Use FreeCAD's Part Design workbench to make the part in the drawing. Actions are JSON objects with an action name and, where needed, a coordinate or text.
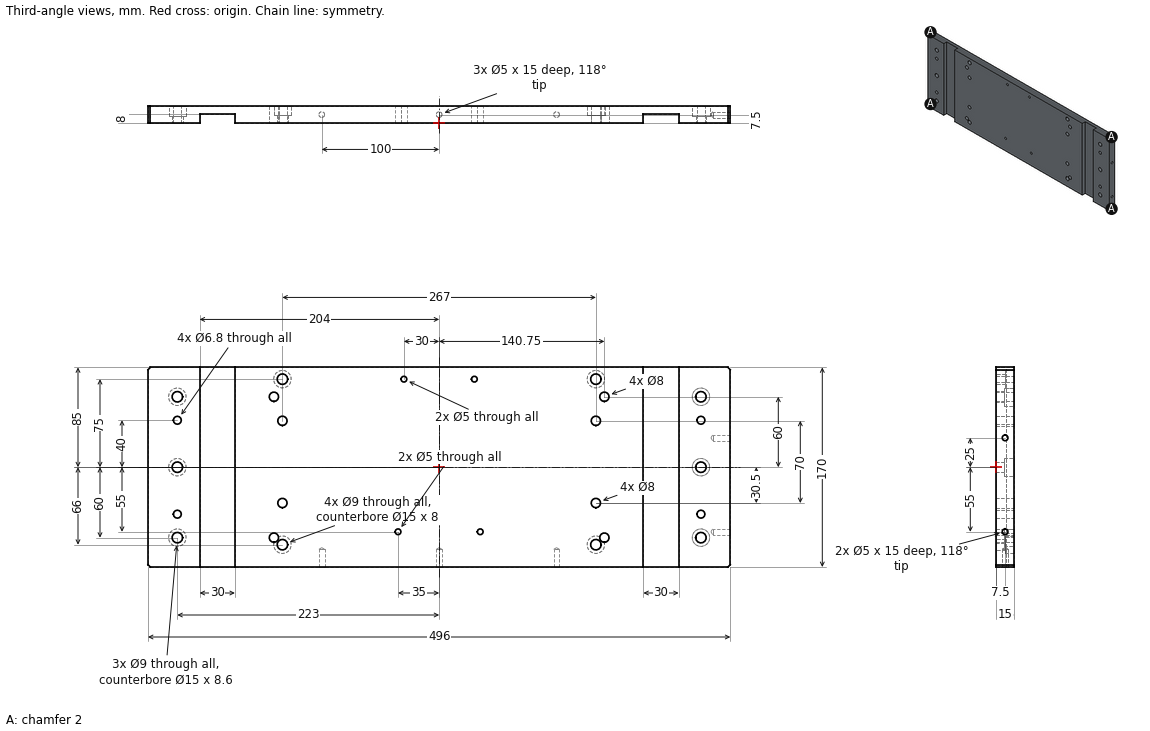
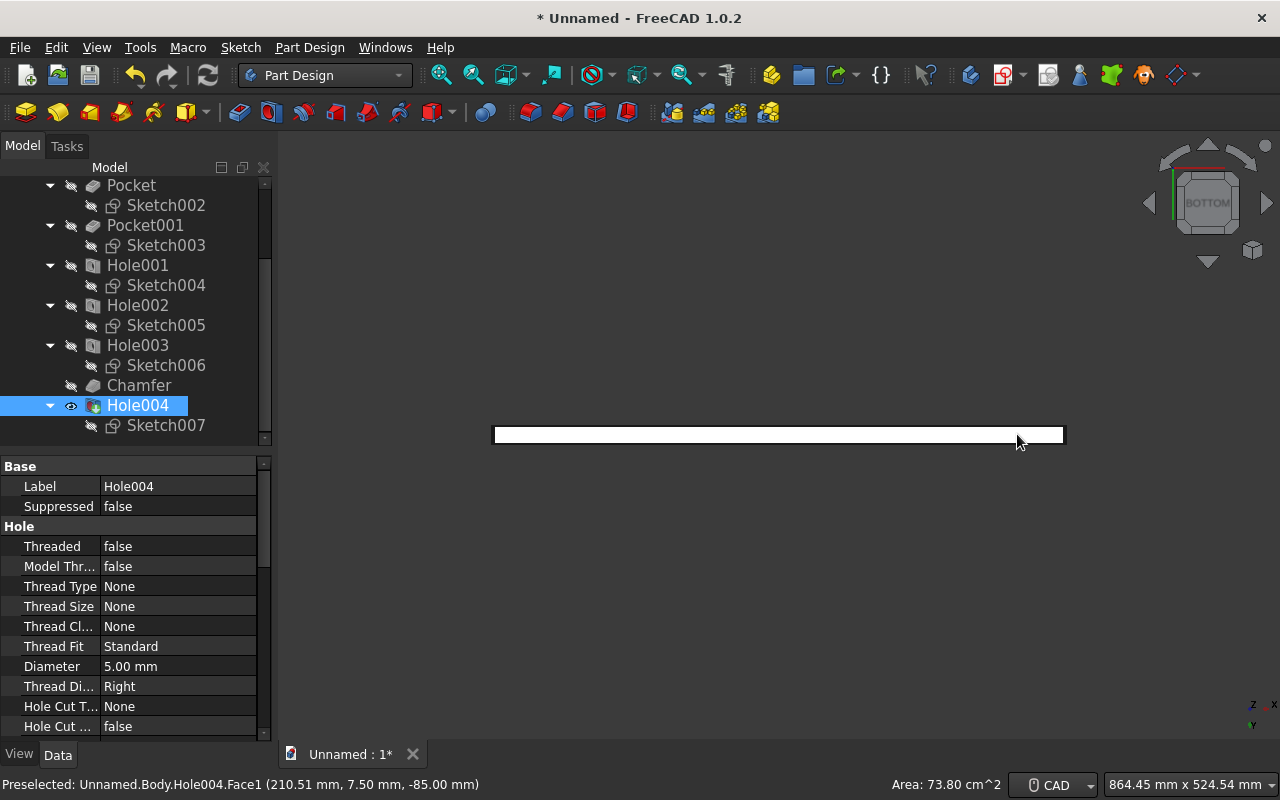
{"action": "left_click", "coordinate": [1004, 76]}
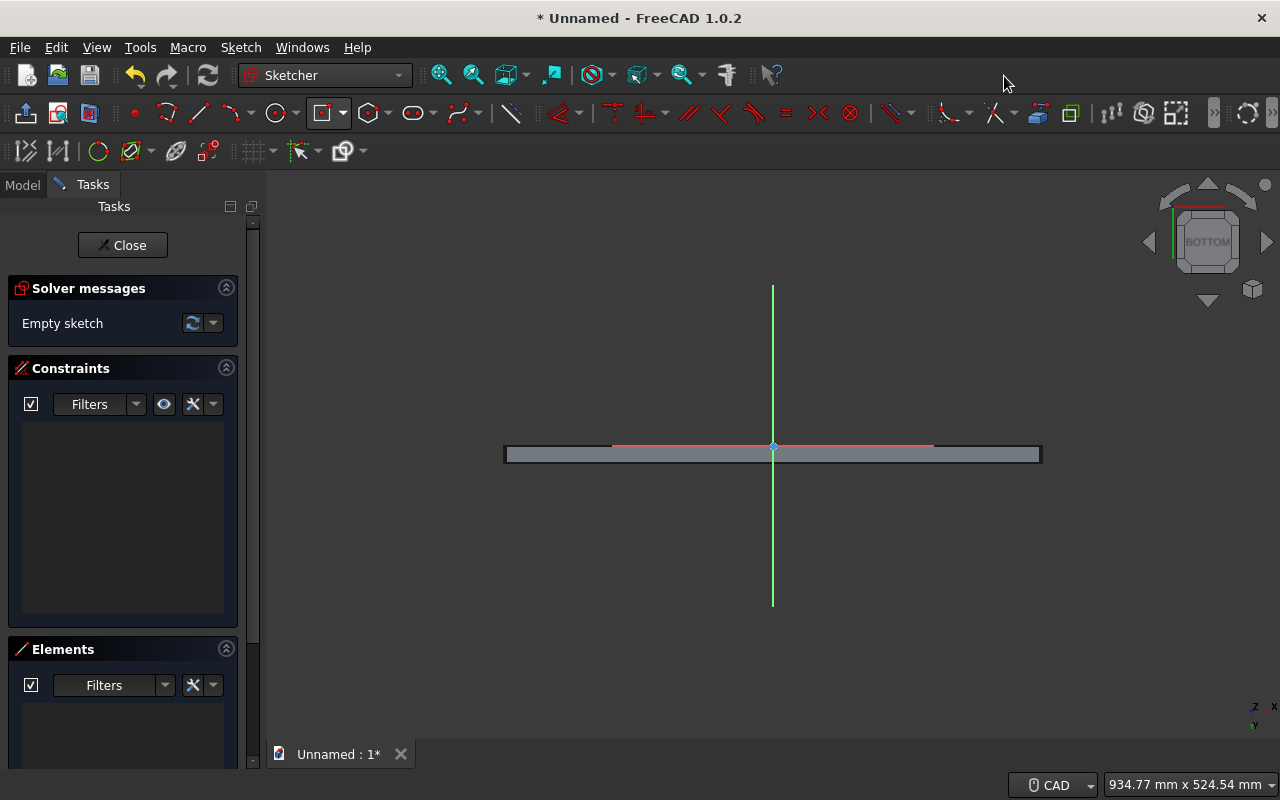
{"action": "scroll", "coordinate": [813, 450], "scroll_direction": "up", "scroll_amount": 5}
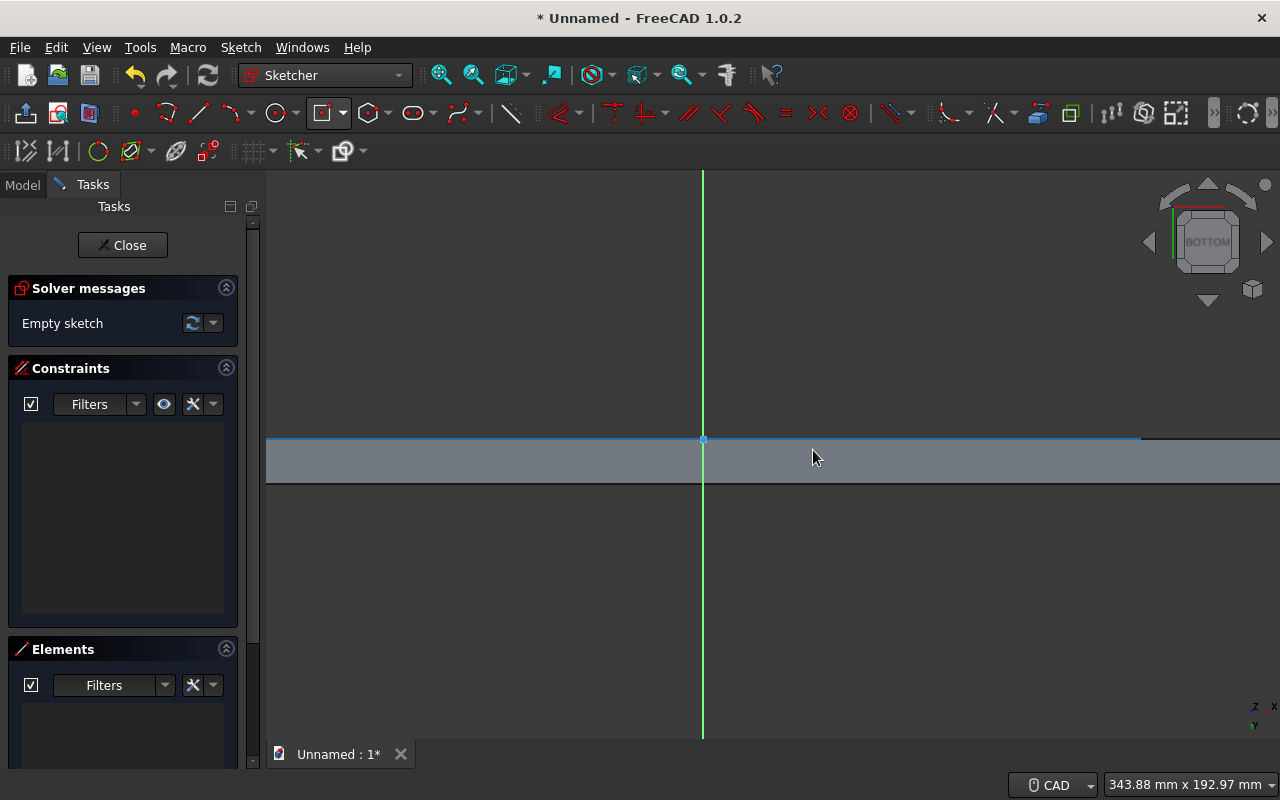
{"action": "left_click", "coordinate": [276, 114]}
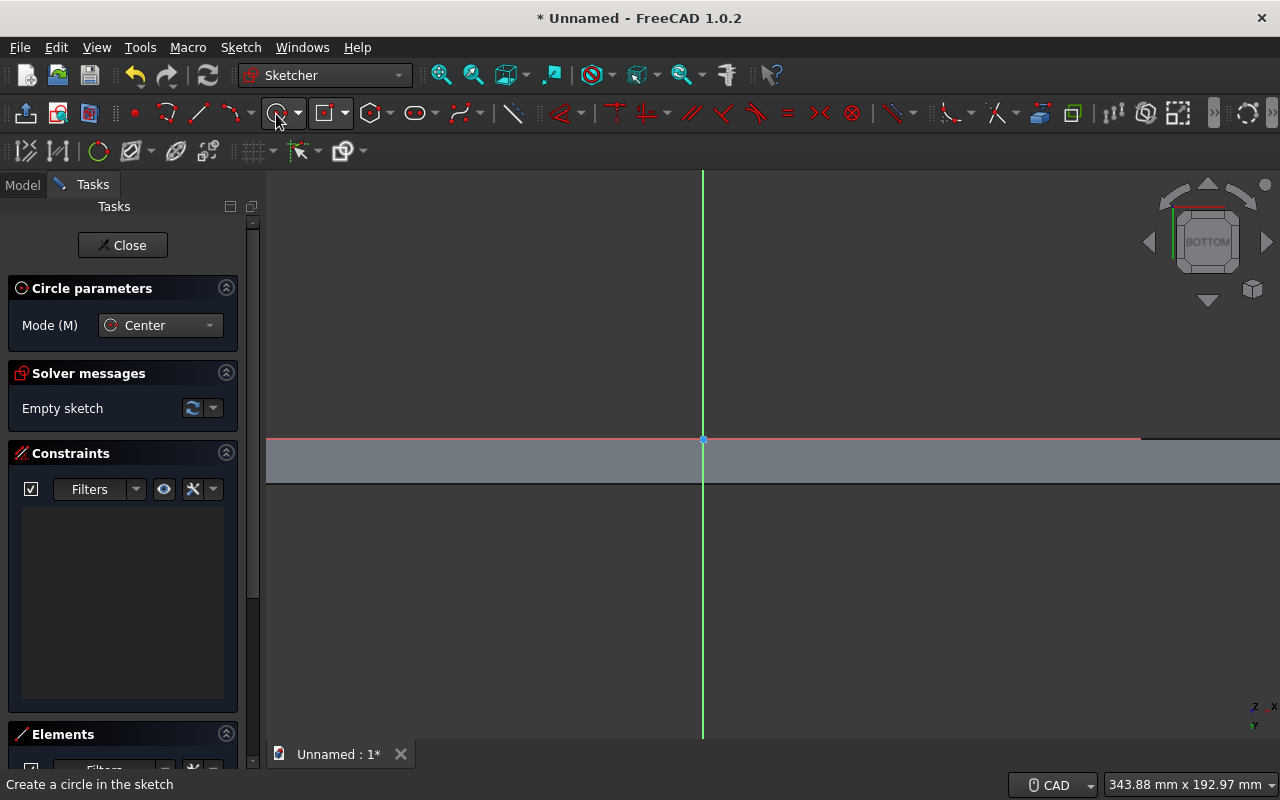
{"action": "scroll", "coordinate": [703, 461], "scroll_direction": "up", "scroll_amount": 6}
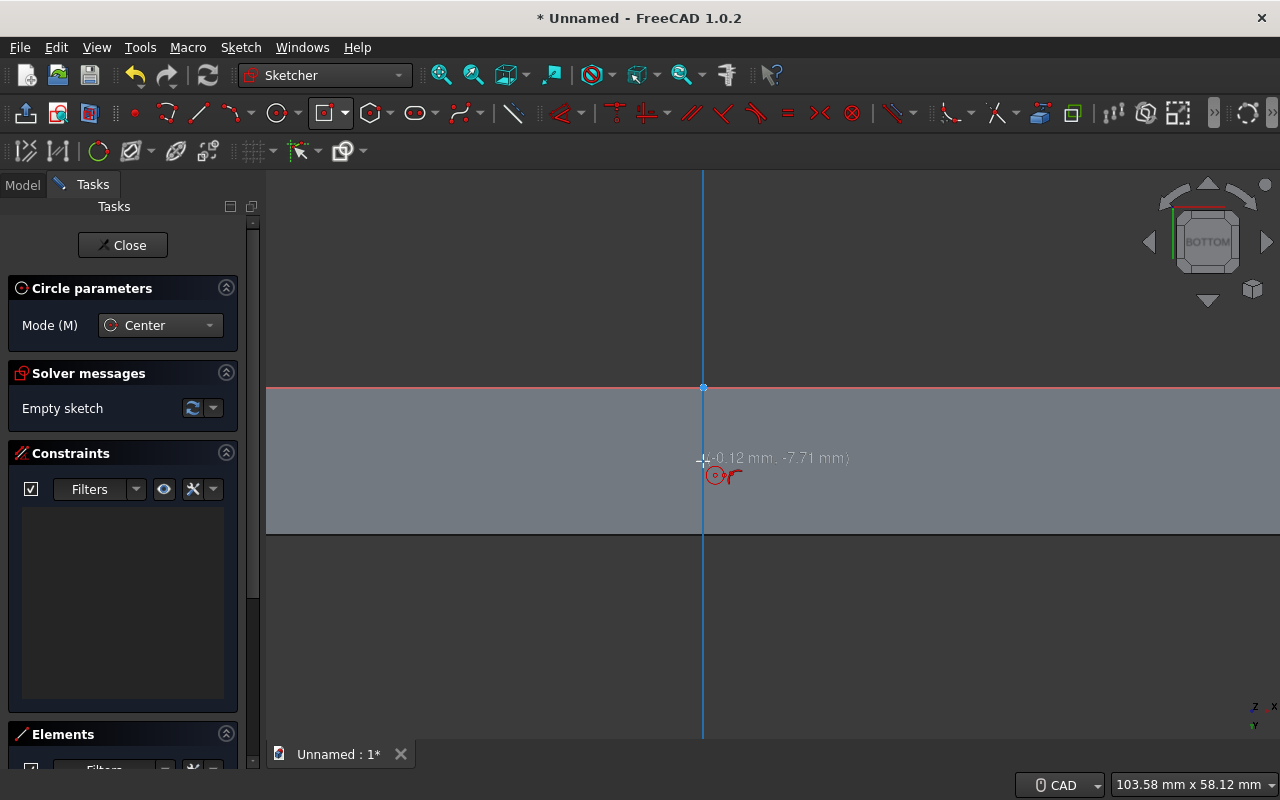
{"action": "left_click", "coordinate": [703, 461]}
{"action": "mouse_move", "coordinate": [720, 444]}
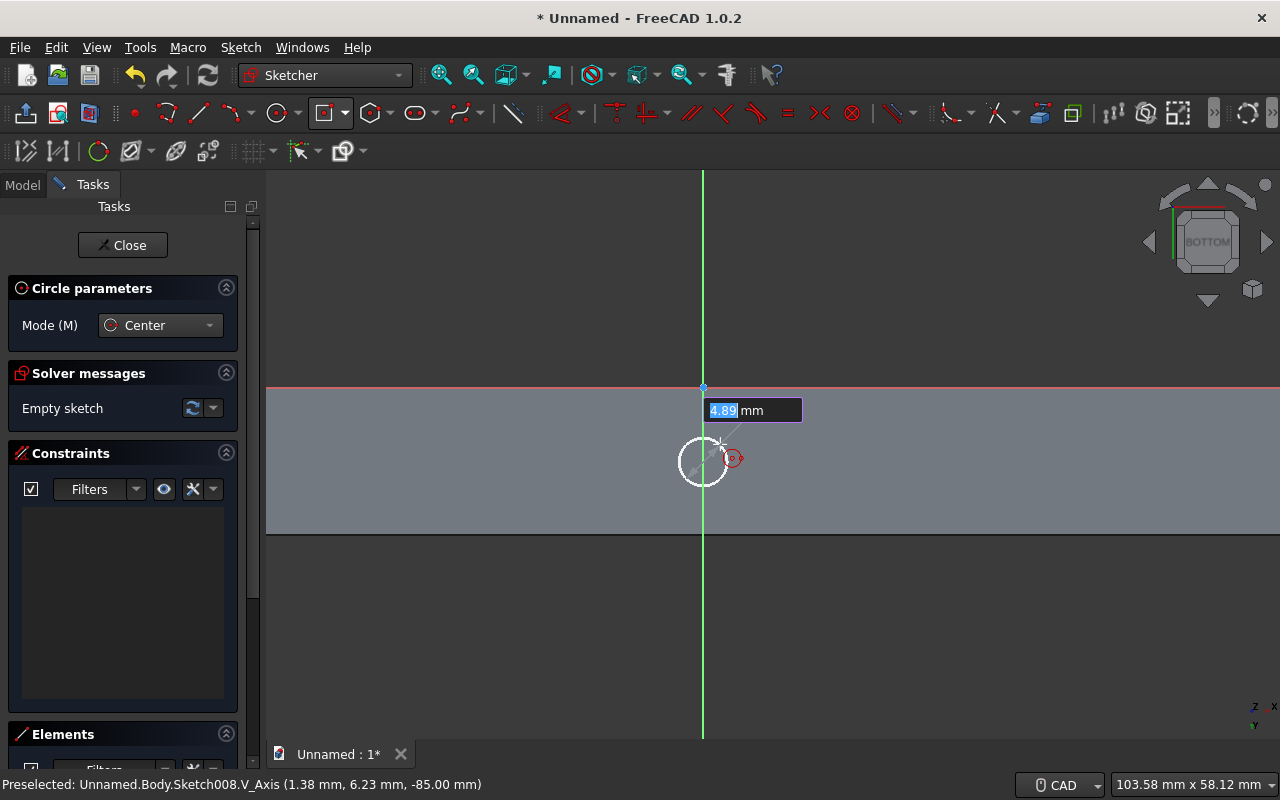
{"action": "type", "text": "5"}
{"action": "key", "text": "Return"}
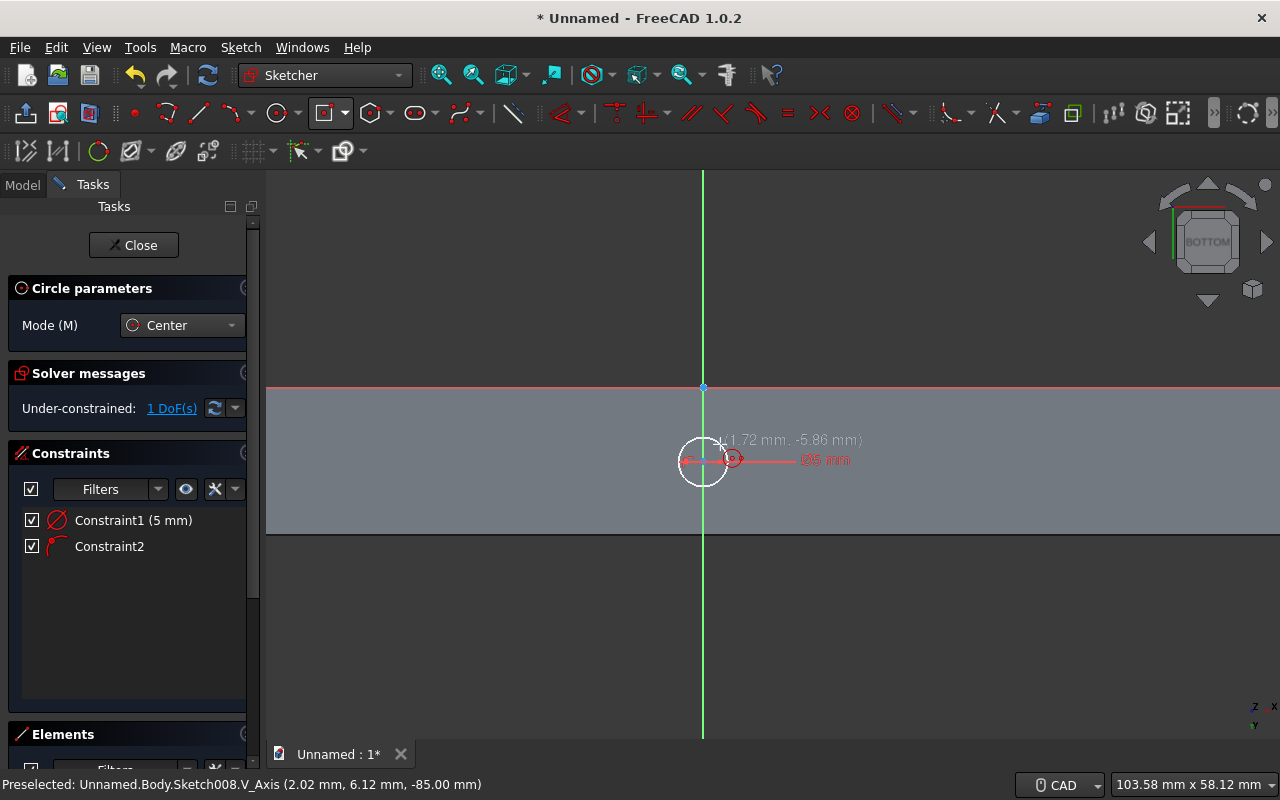
{"action": "scroll", "coordinate": [705, 462], "scroll_direction": "down", "scroll_amount": 6}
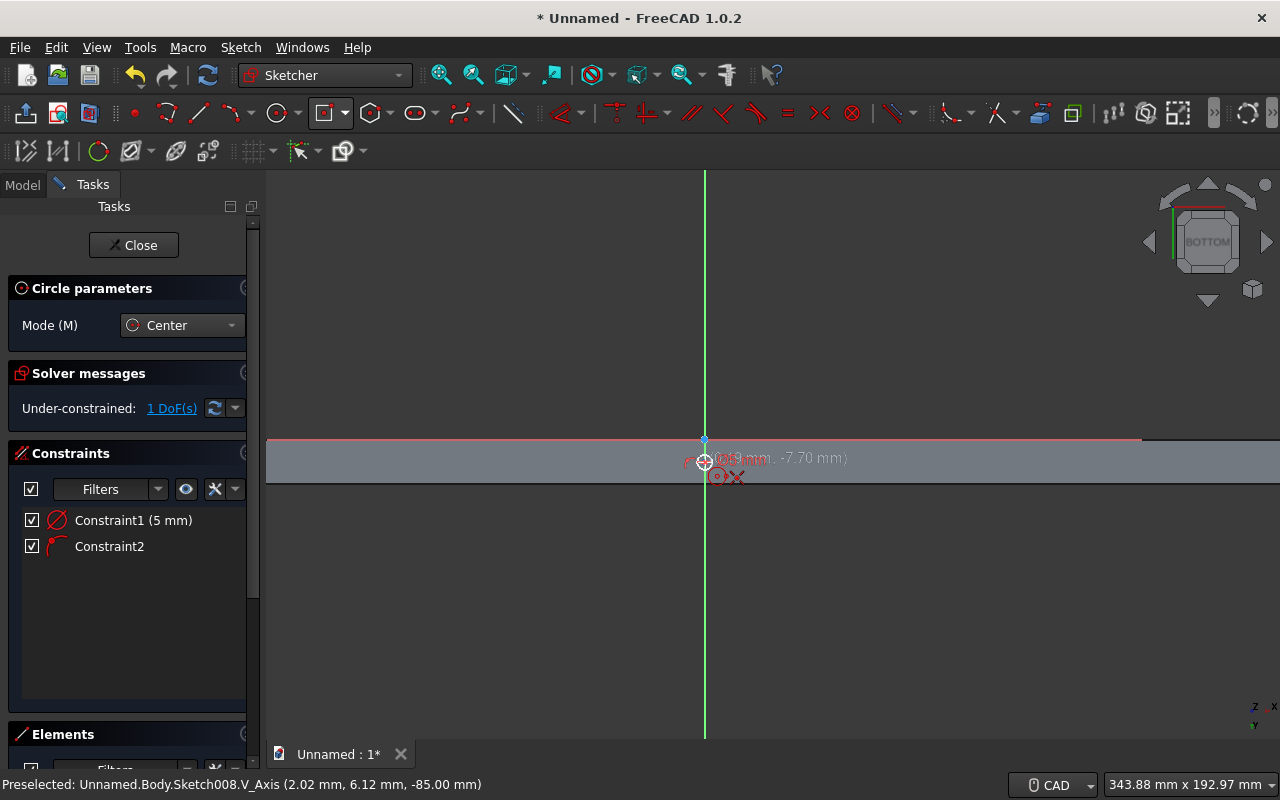
{"action": "scroll", "coordinate": [410, 462], "scroll_direction": "up", "scroll_amount": 6}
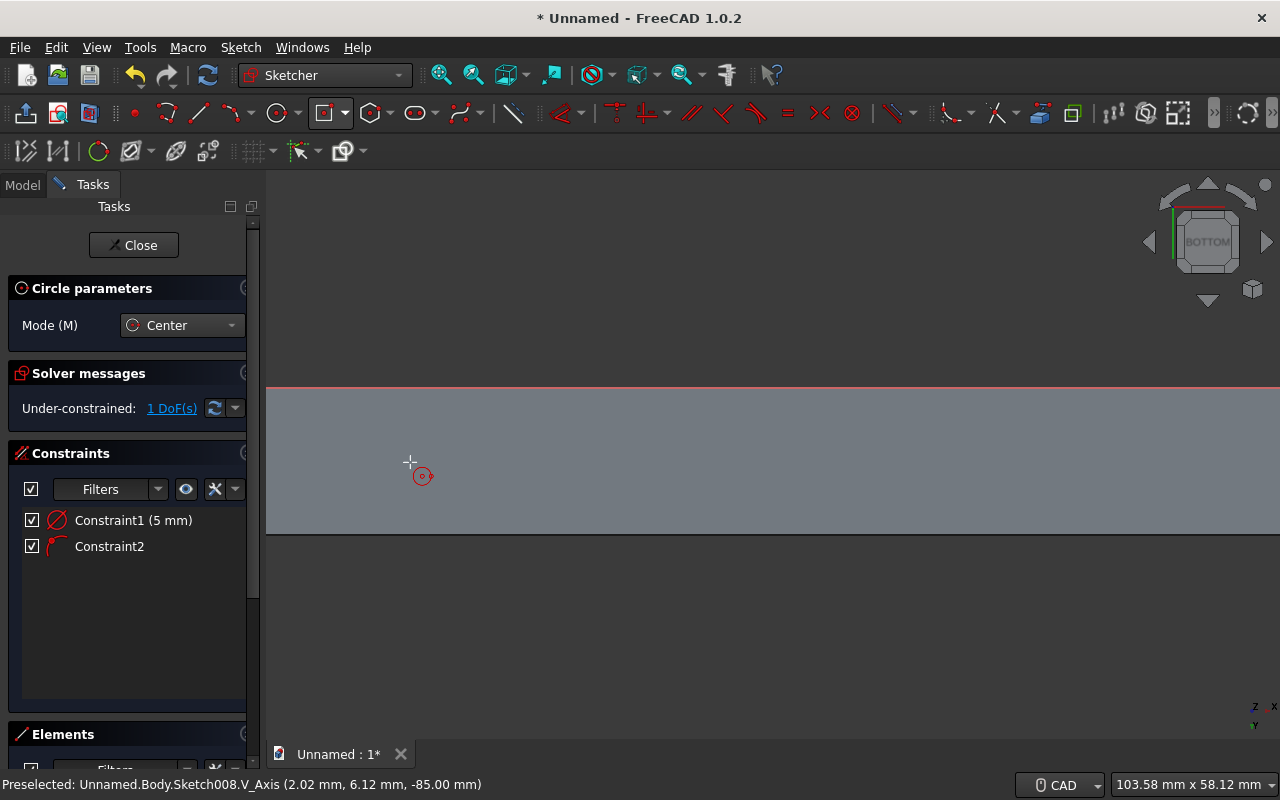
{"action": "left_click", "coordinate": [409, 461]}
{"action": "mouse_move", "coordinate": [427, 444]}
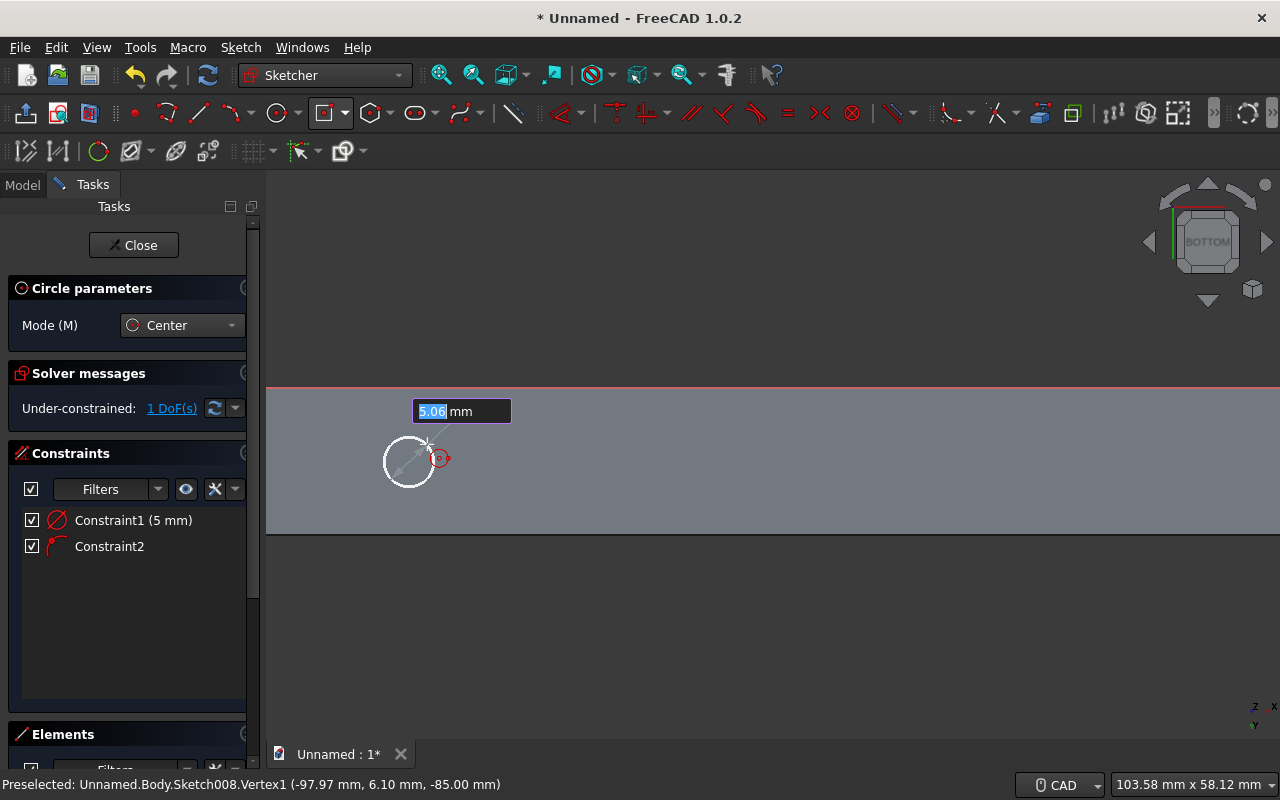
{"action": "type", "text": "5"}
{"action": "key", "text": "Return"}